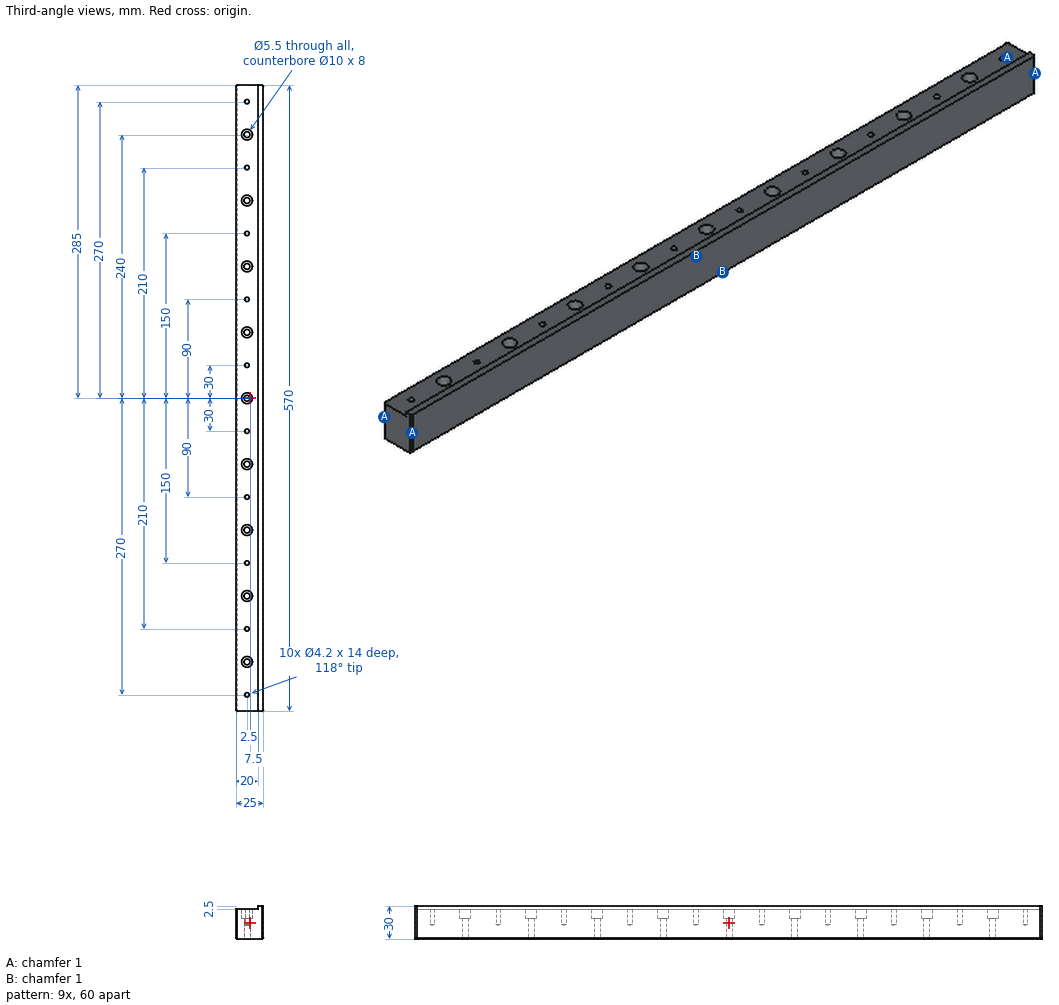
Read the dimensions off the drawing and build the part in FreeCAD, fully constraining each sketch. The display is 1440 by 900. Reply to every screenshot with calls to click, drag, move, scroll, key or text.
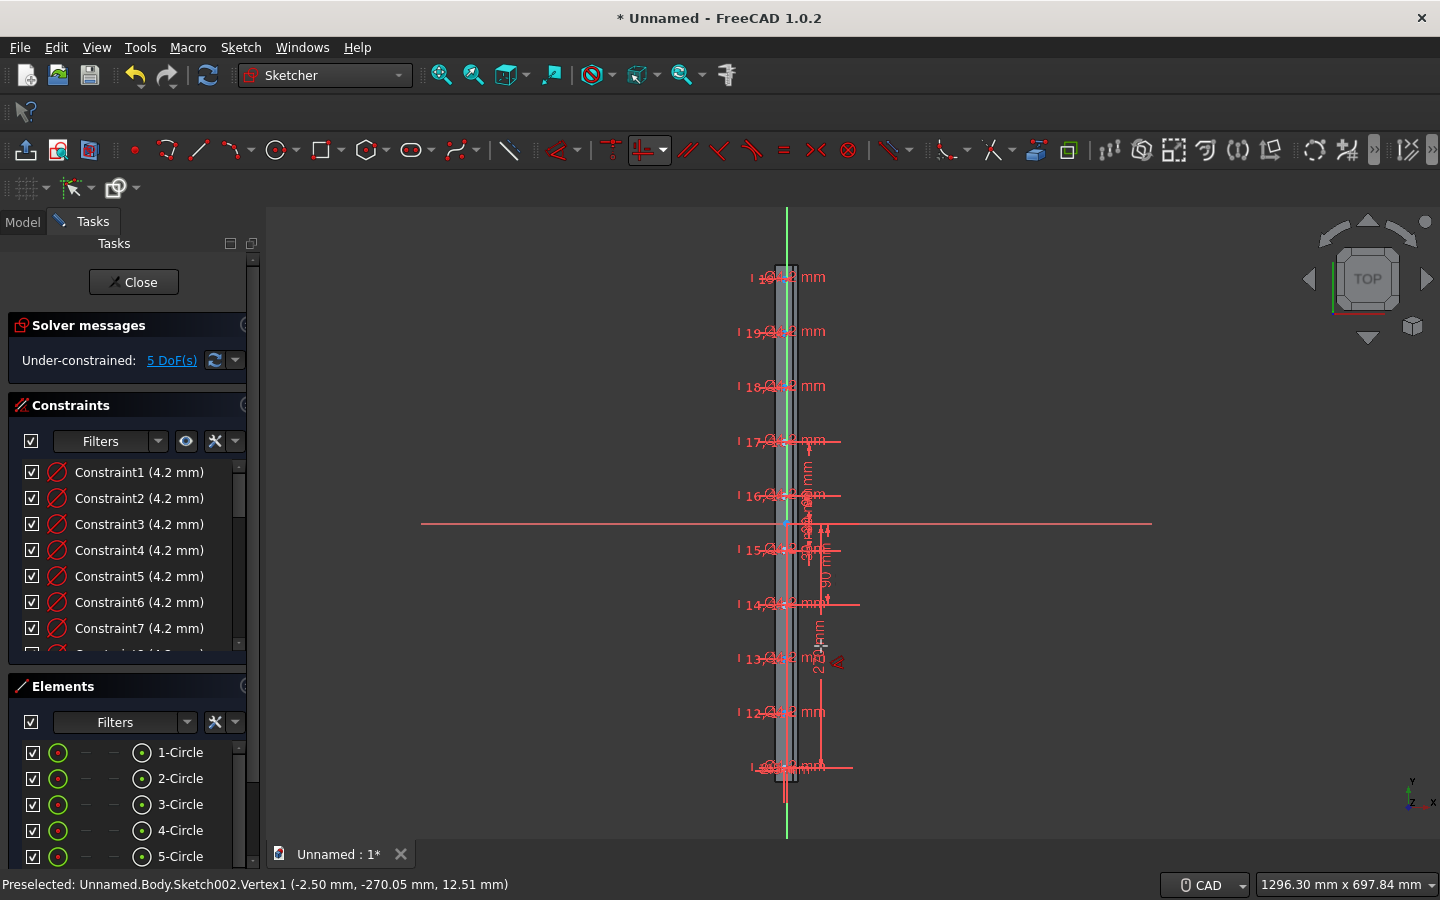
click(784, 714)
click(821, 619)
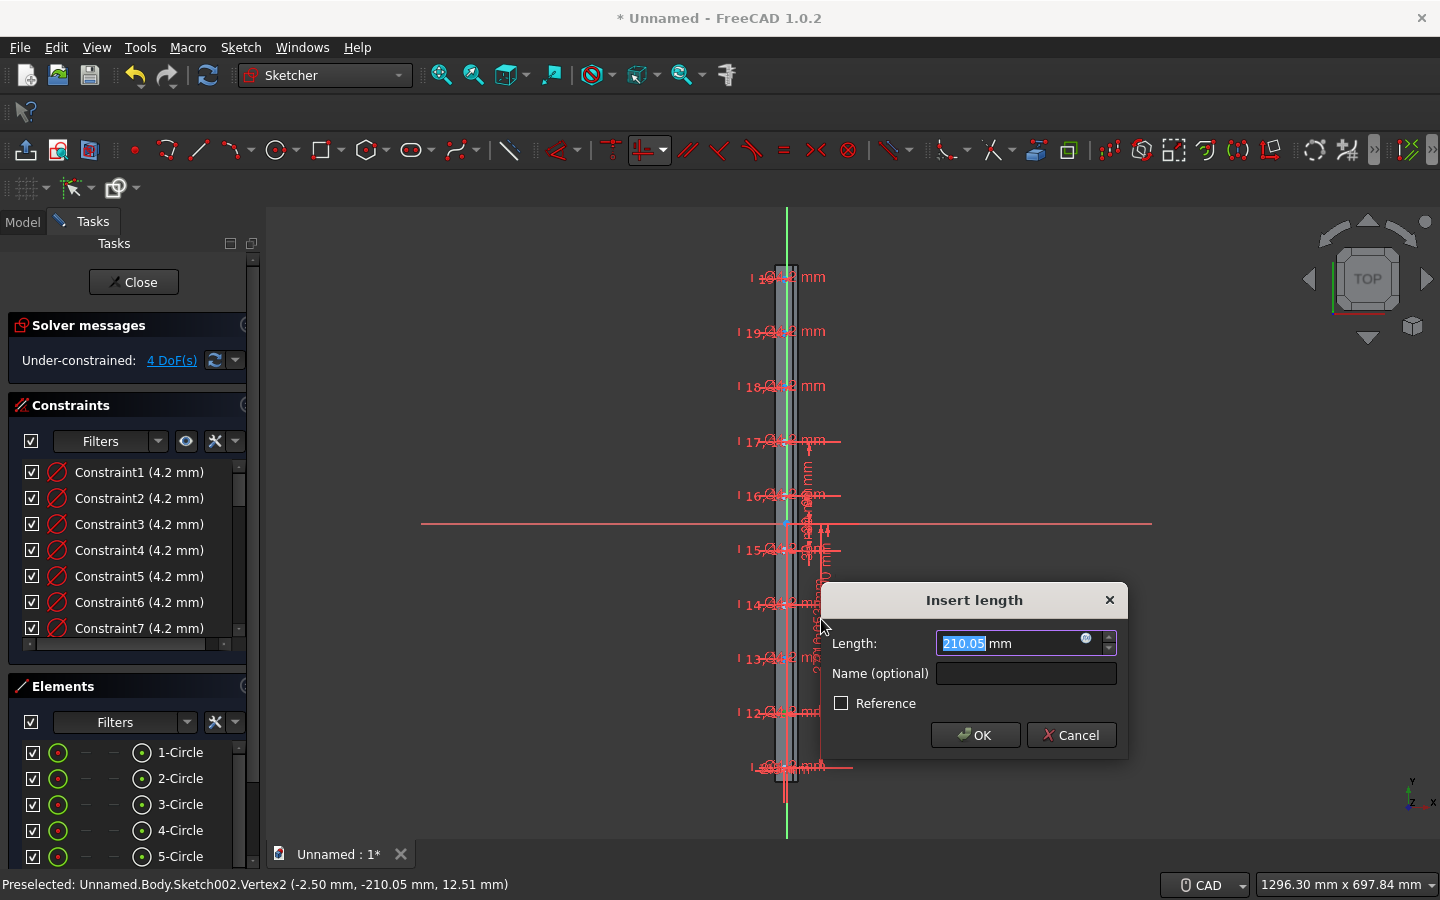
text(210)
key(Return)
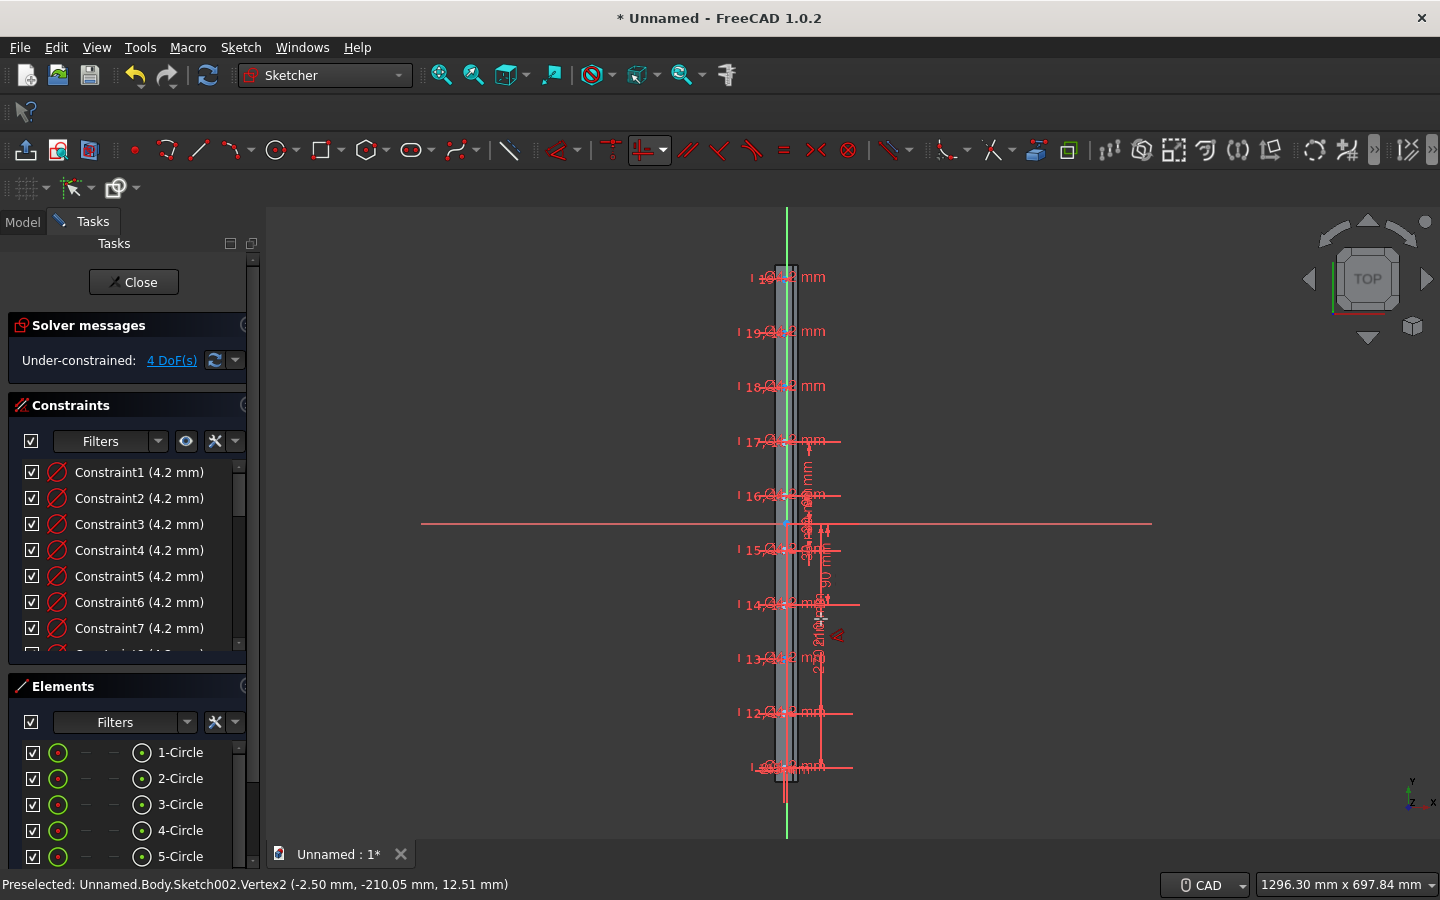
click(784, 659)
click(821, 592)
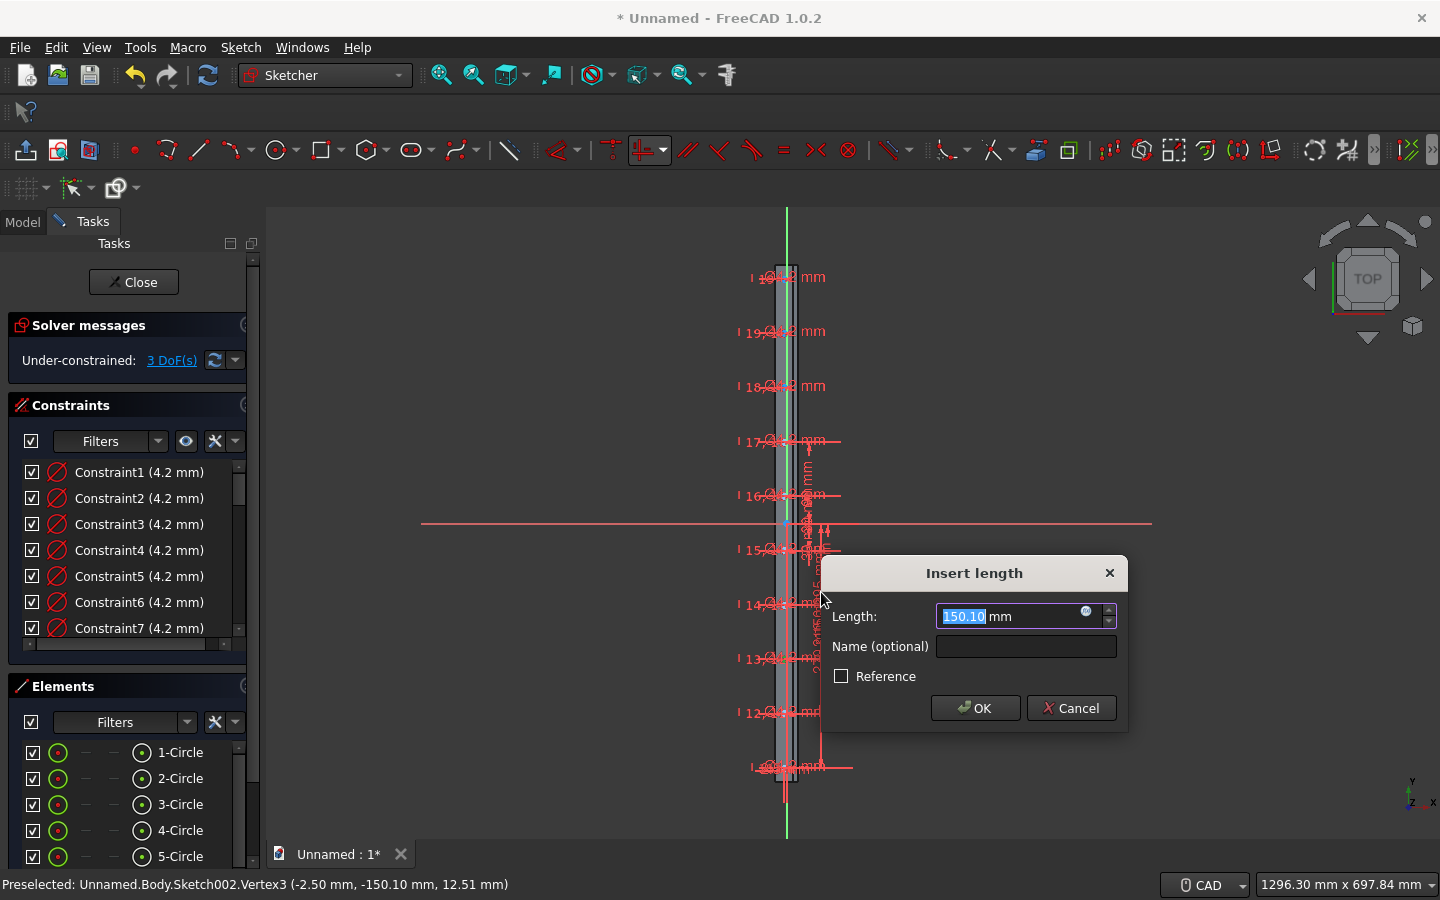
text(150)
key(Return)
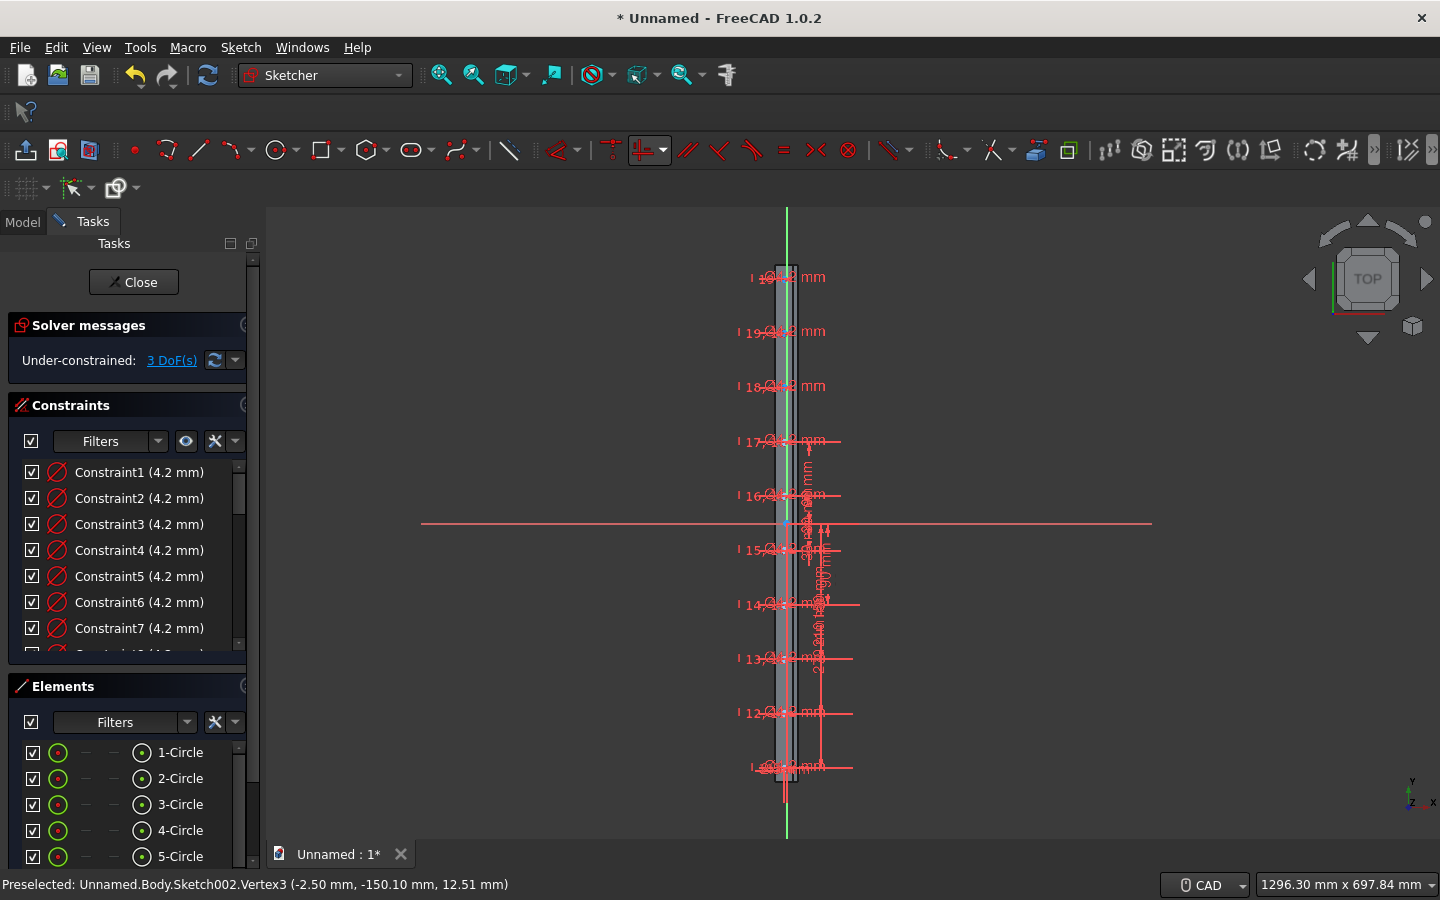
click(784, 388)
click(821, 456)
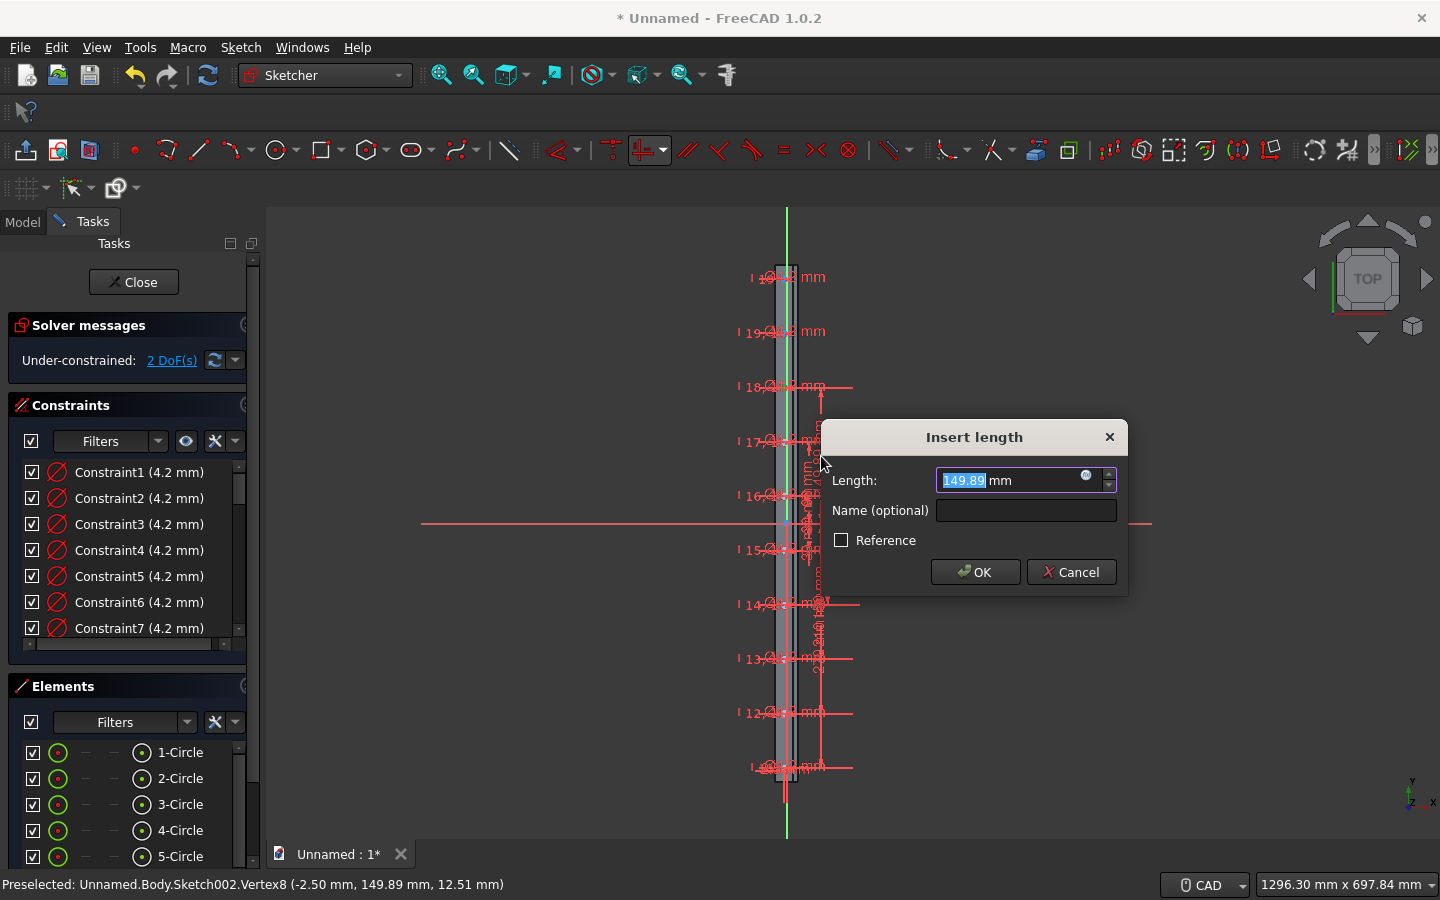
text(150)
key(Return)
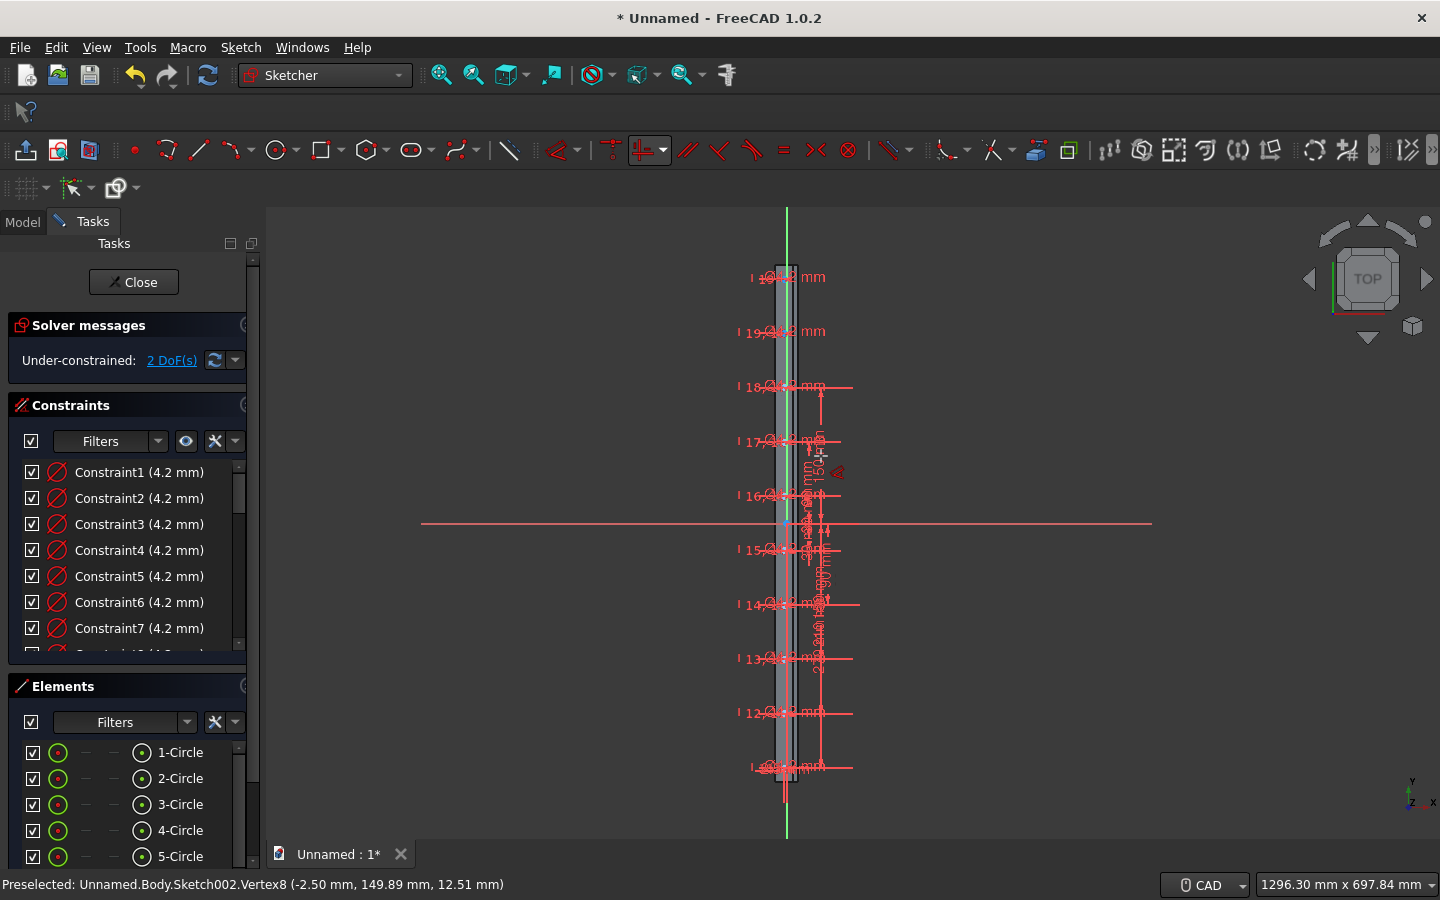
click(784, 333)
click(821, 428)